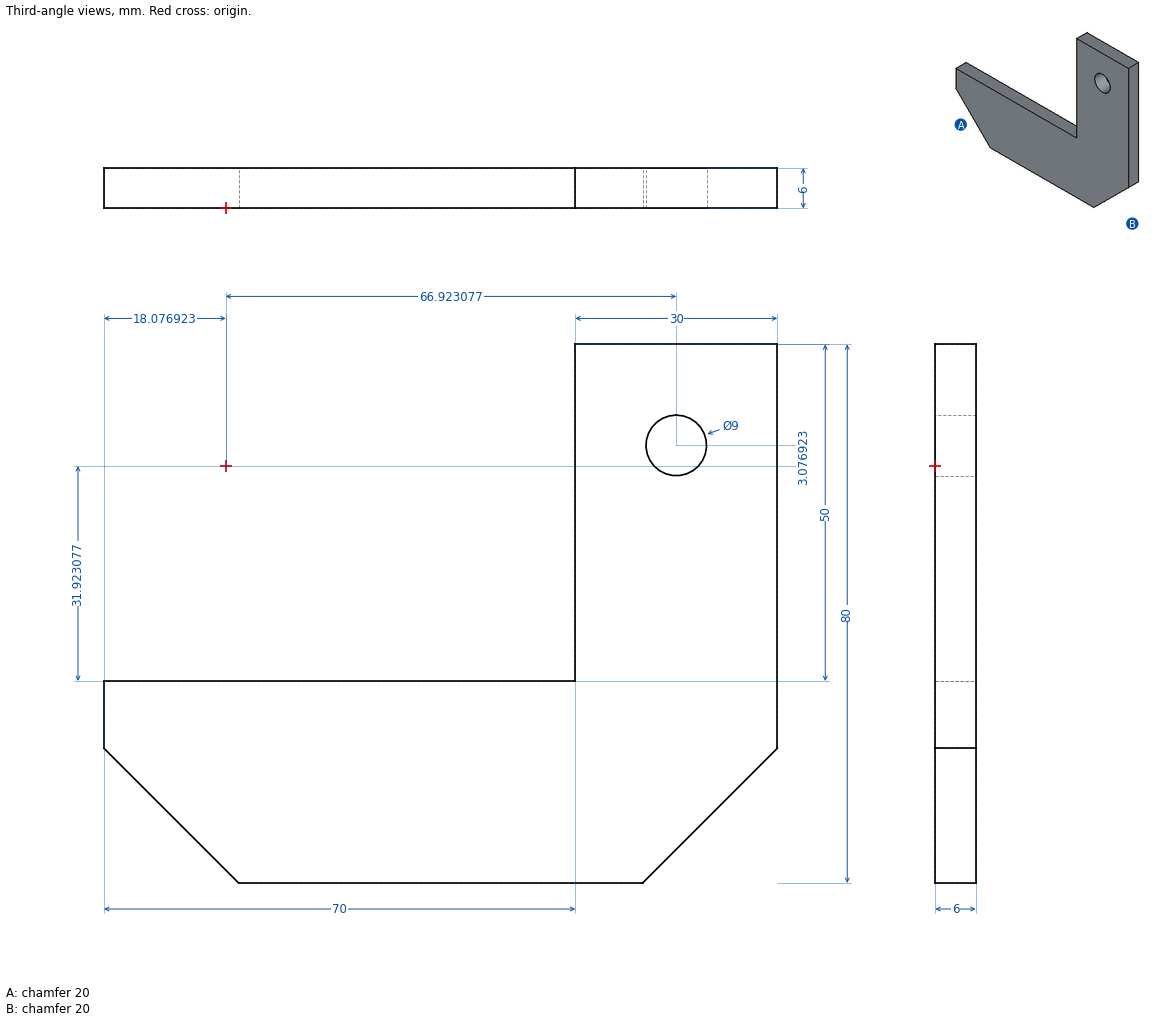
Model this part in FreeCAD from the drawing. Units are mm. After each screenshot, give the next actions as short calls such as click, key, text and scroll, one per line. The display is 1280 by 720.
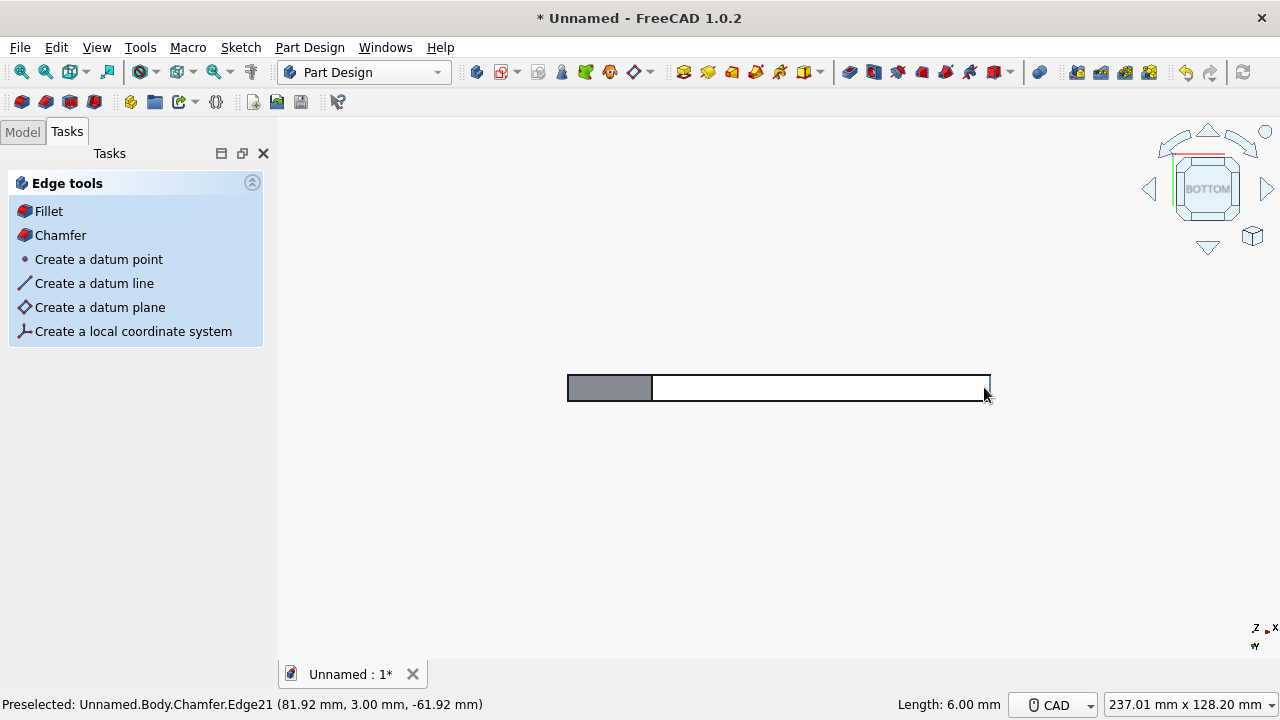
click(46, 102)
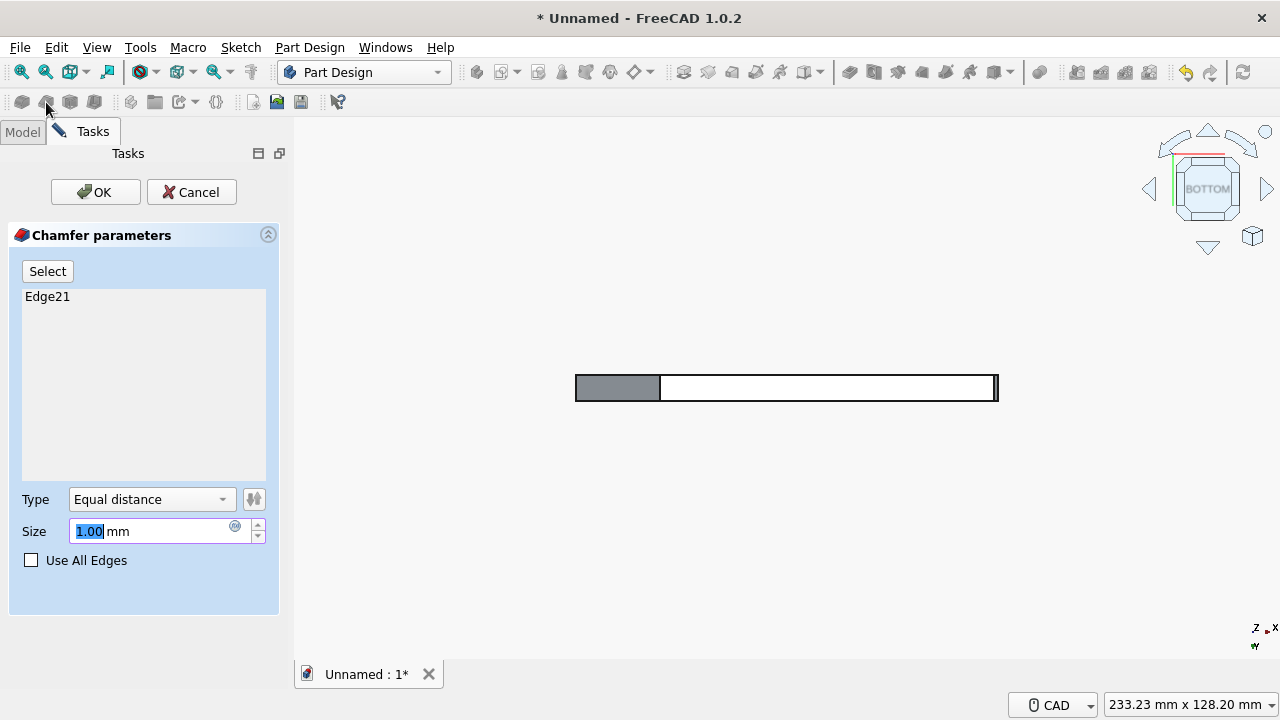
text(20)
key(Tab)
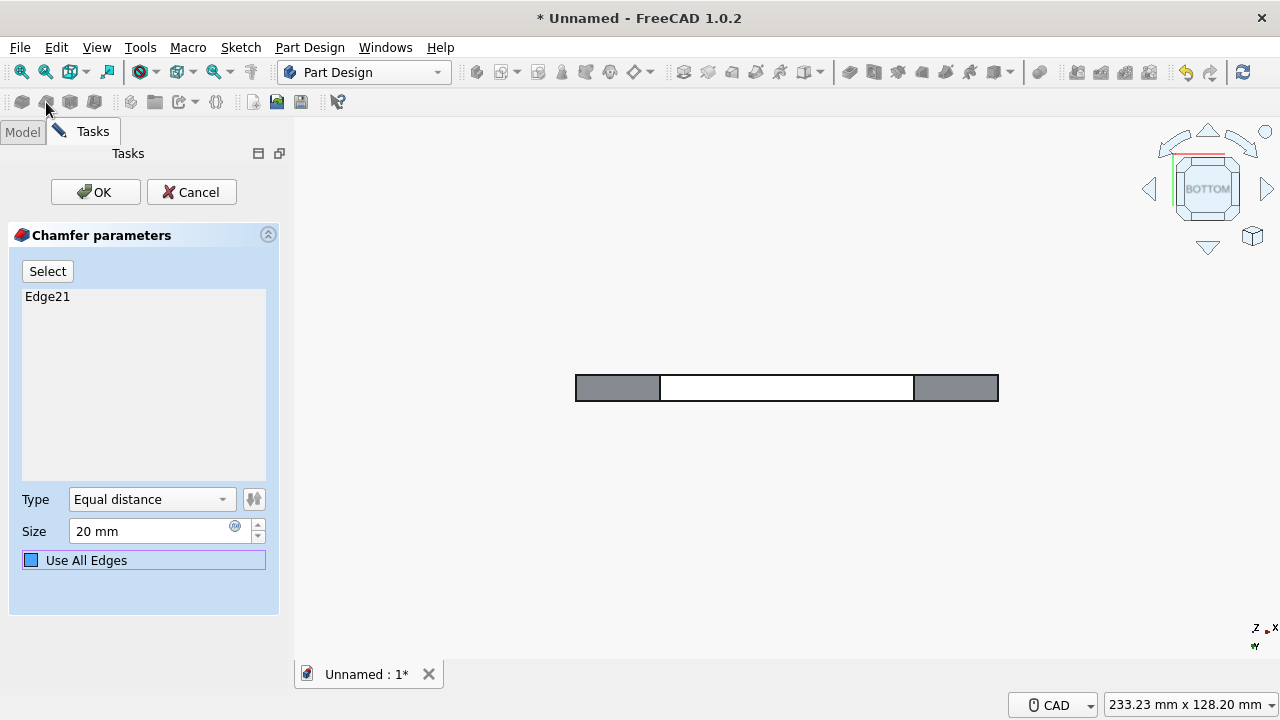
click(96, 192)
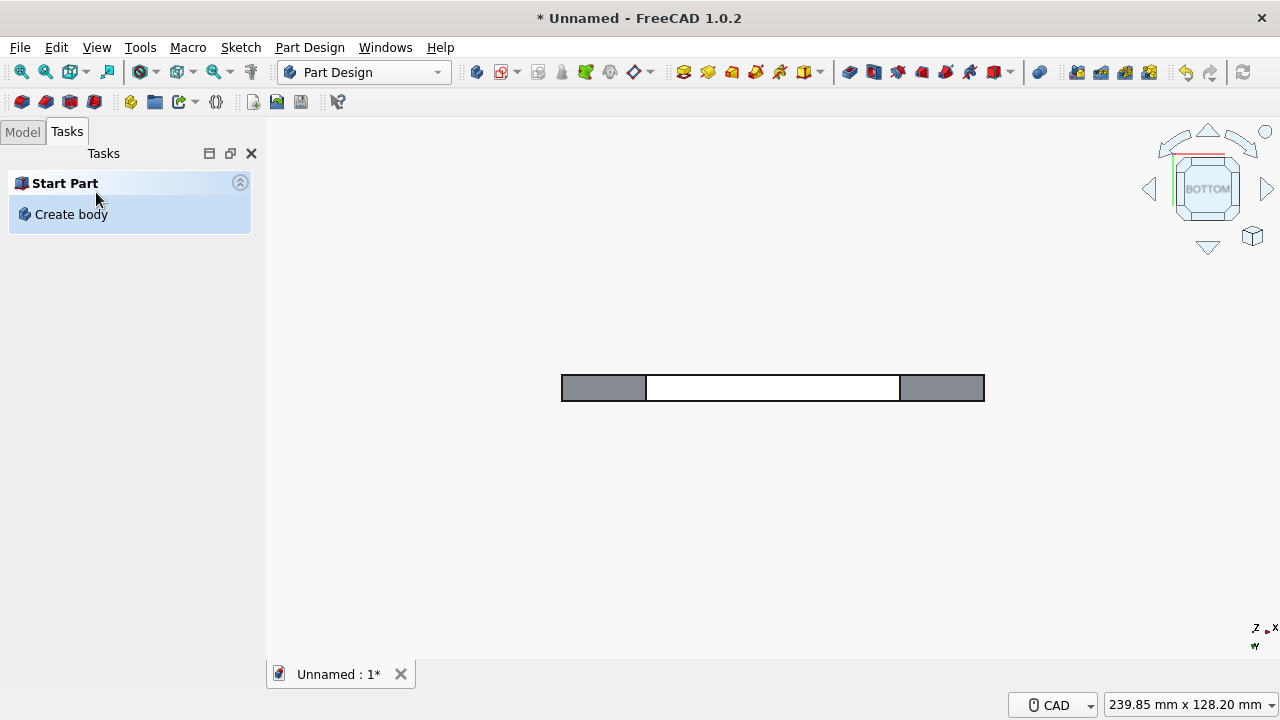
key(0)